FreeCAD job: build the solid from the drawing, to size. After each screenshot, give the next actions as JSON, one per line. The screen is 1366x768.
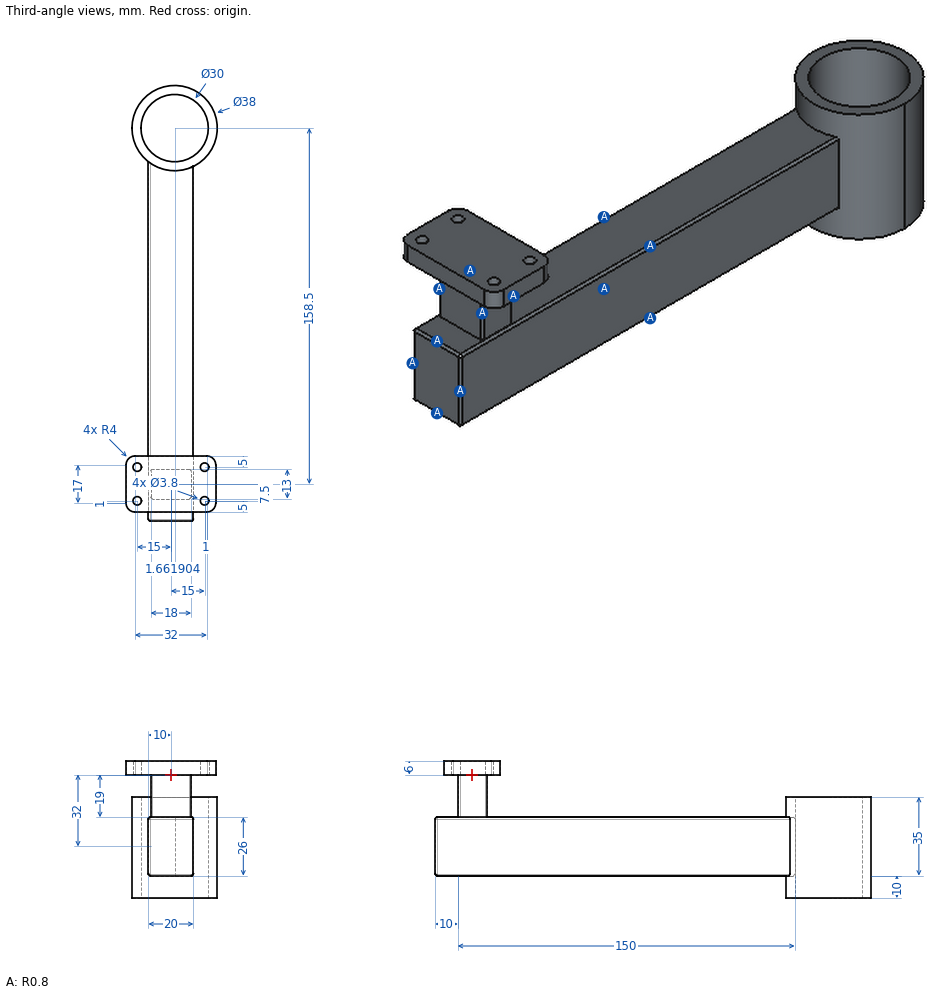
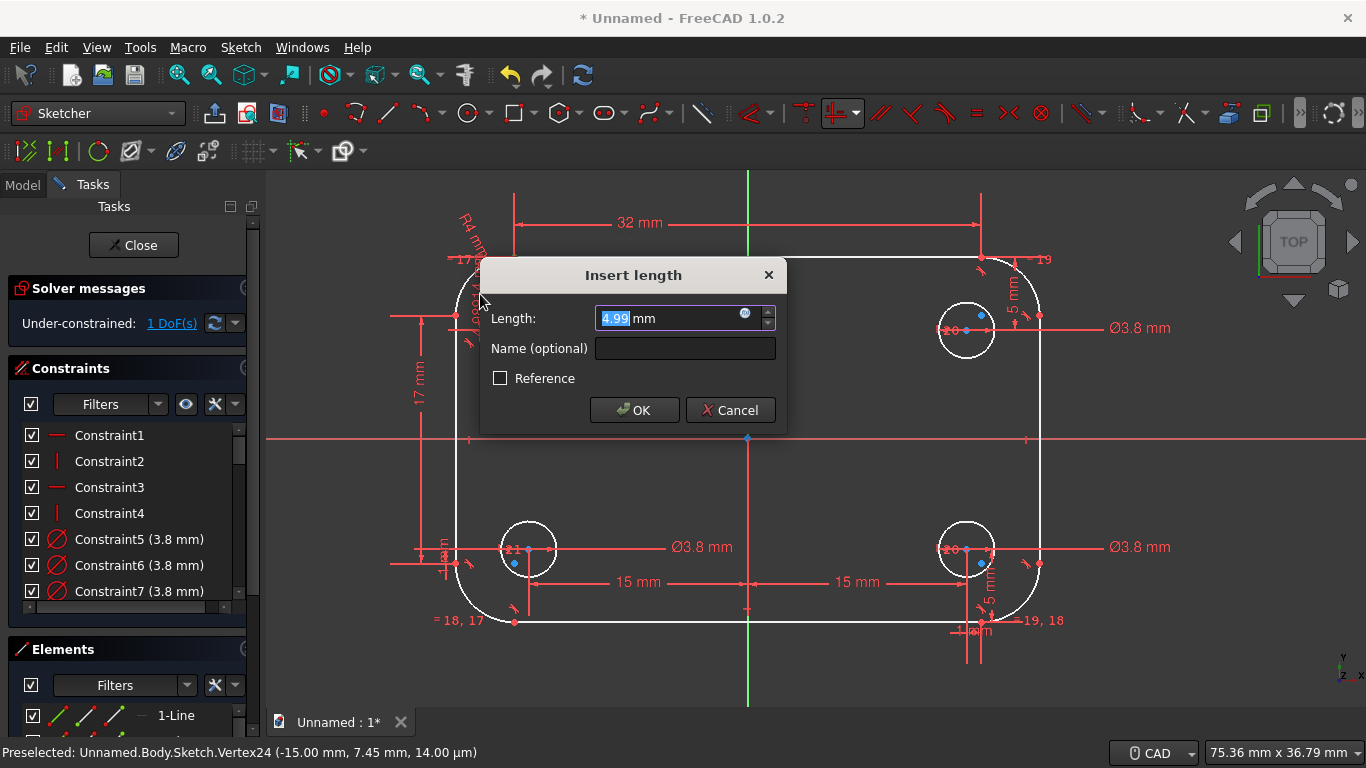
{"action": "type", "text": "5"}
{"action": "key", "text": "Return"}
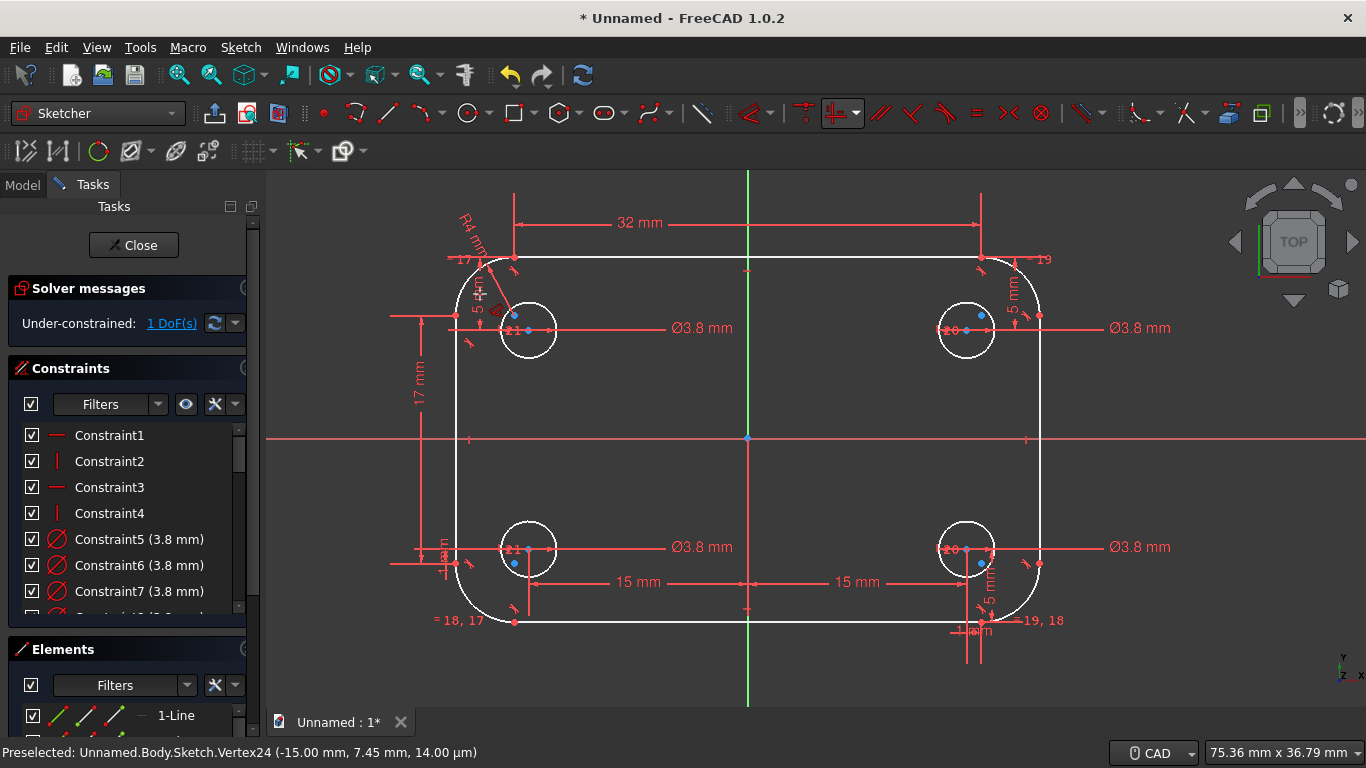
{"action": "left_click", "coordinate": [967, 549]}
{"action": "left_click", "coordinate": [1001, 494]}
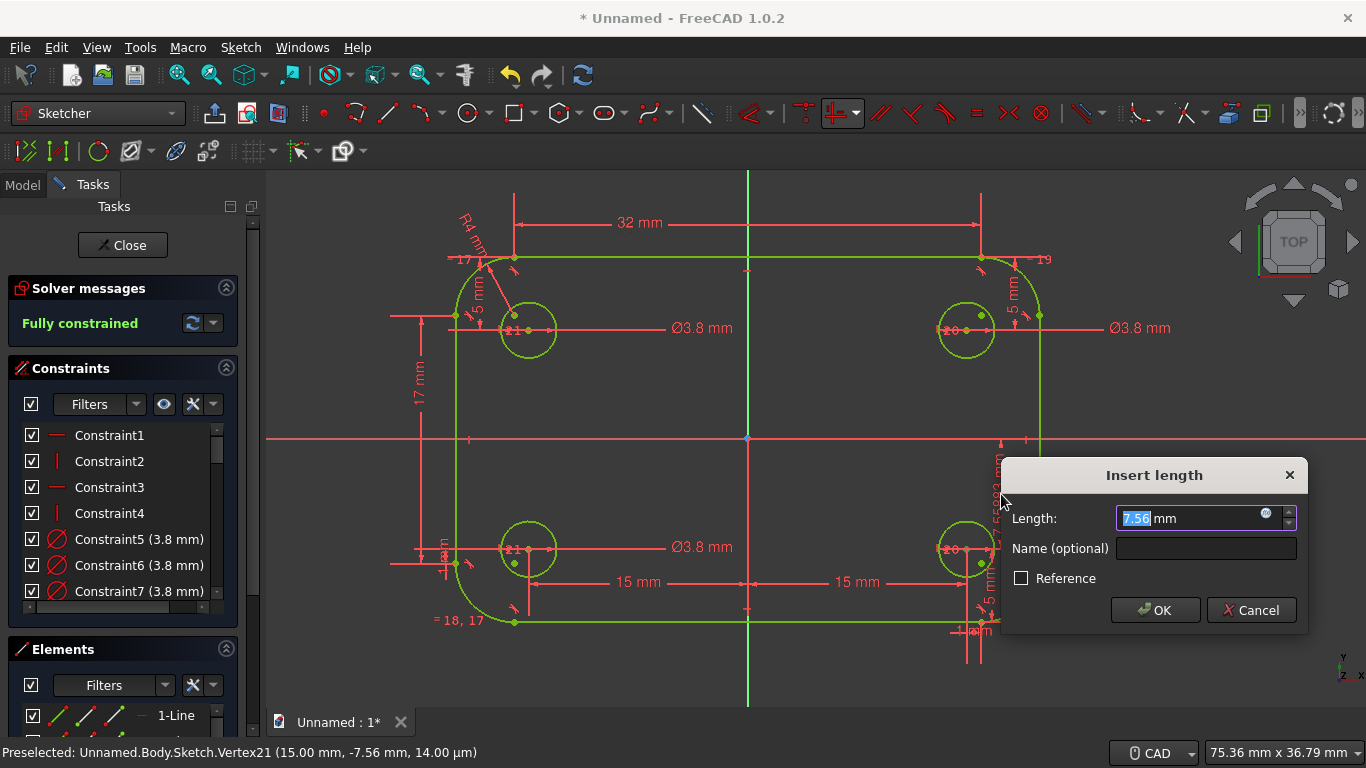
{"action": "type", "text": "7.5"}
{"action": "key", "text": "Return"}
{"action": "key", "text": "Escape"}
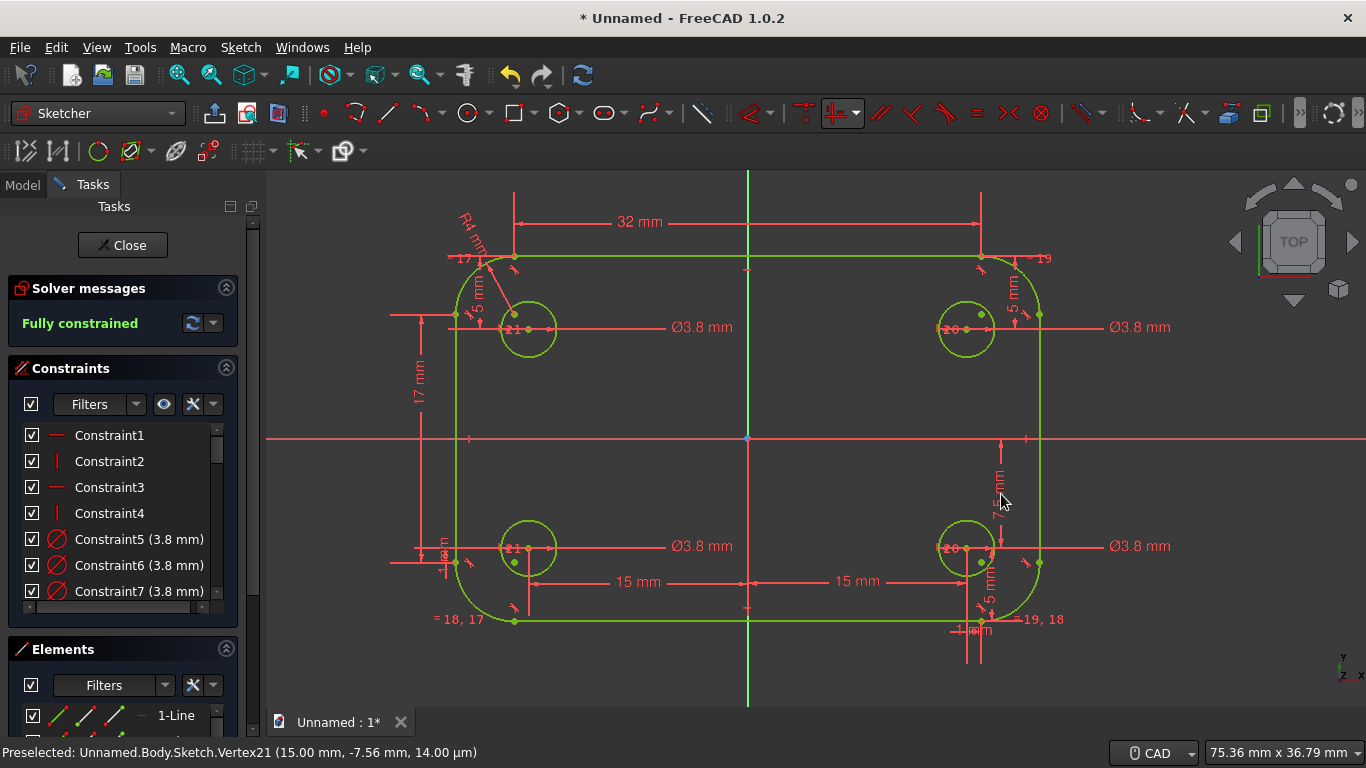
{"action": "left_click", "coordinate": [123, 245]}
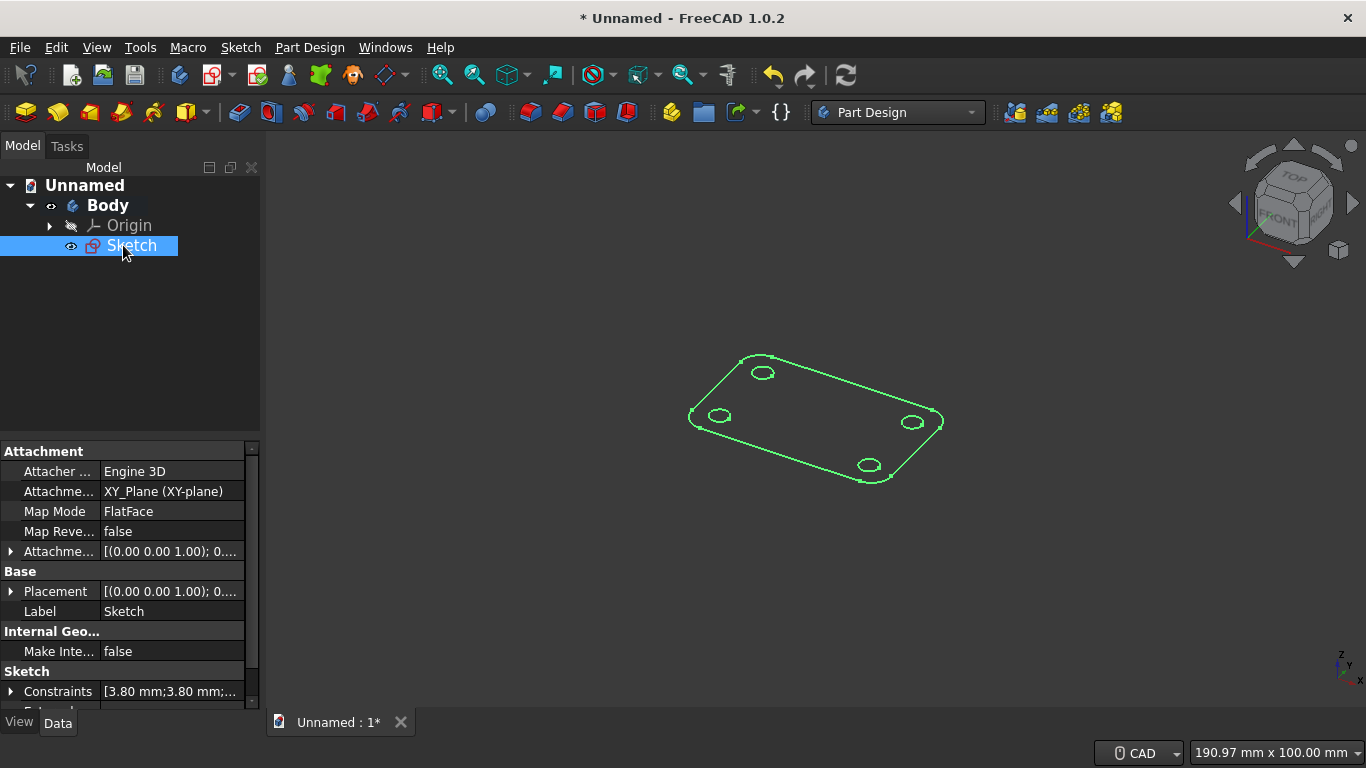
{"action": "left_click", "coordinate": [26, 112]}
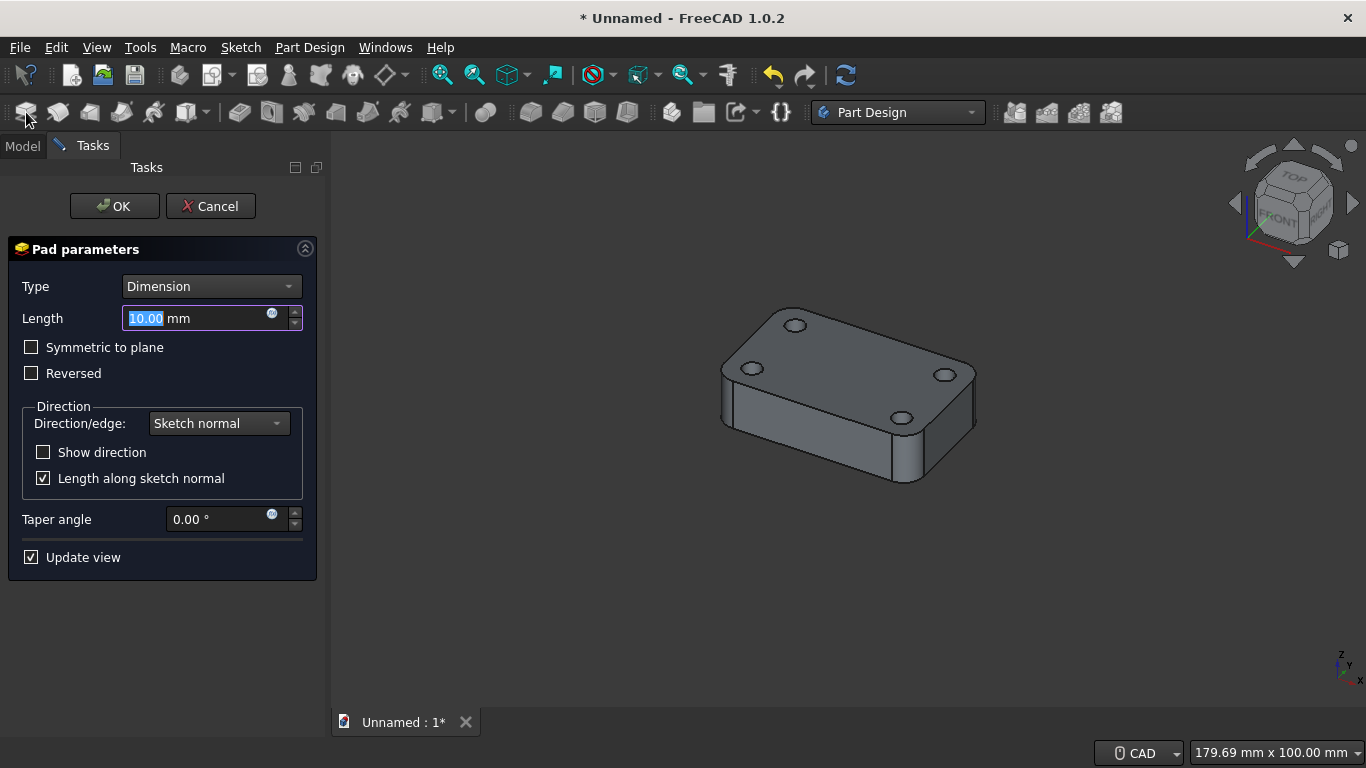
{"action": "type", "text": "6"}
{"action": "key", "text": "Tab"}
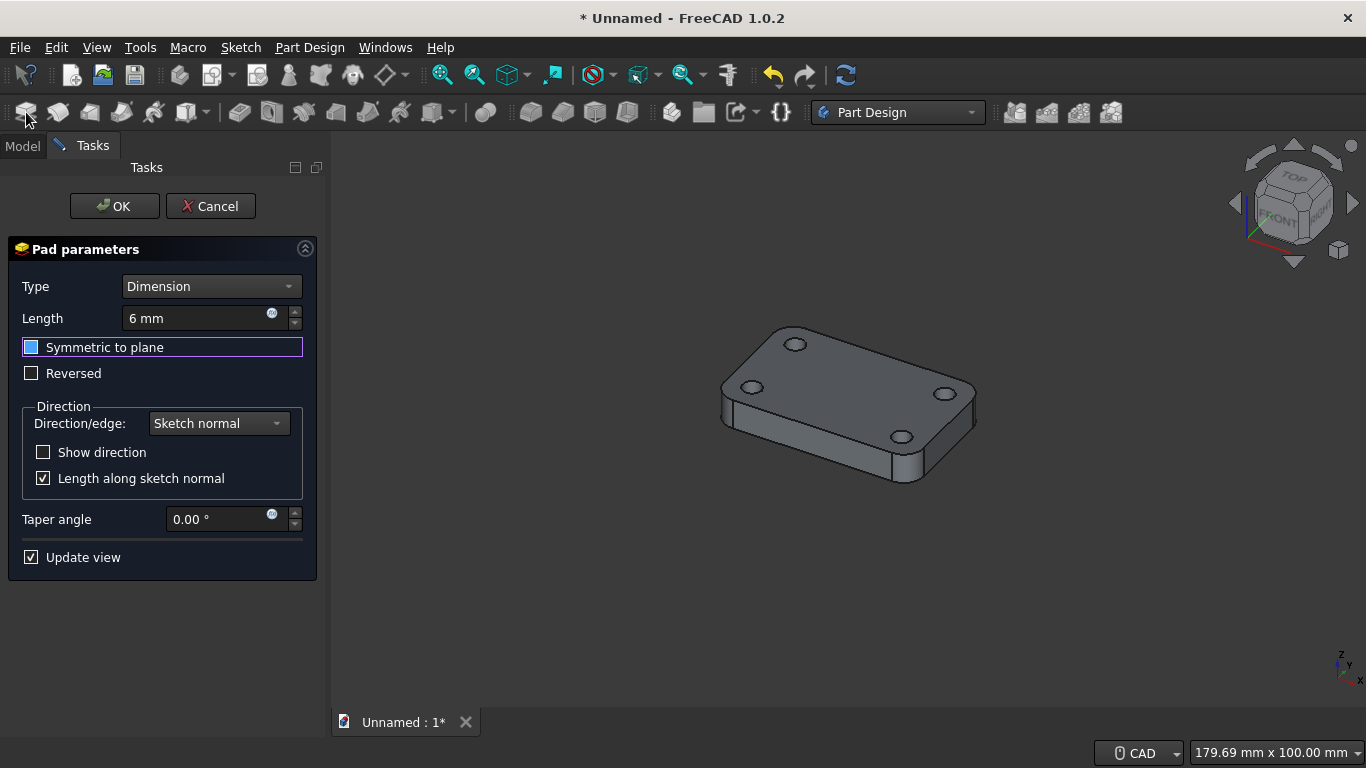
{"action": "left_click", "coordinate": [115, 206]}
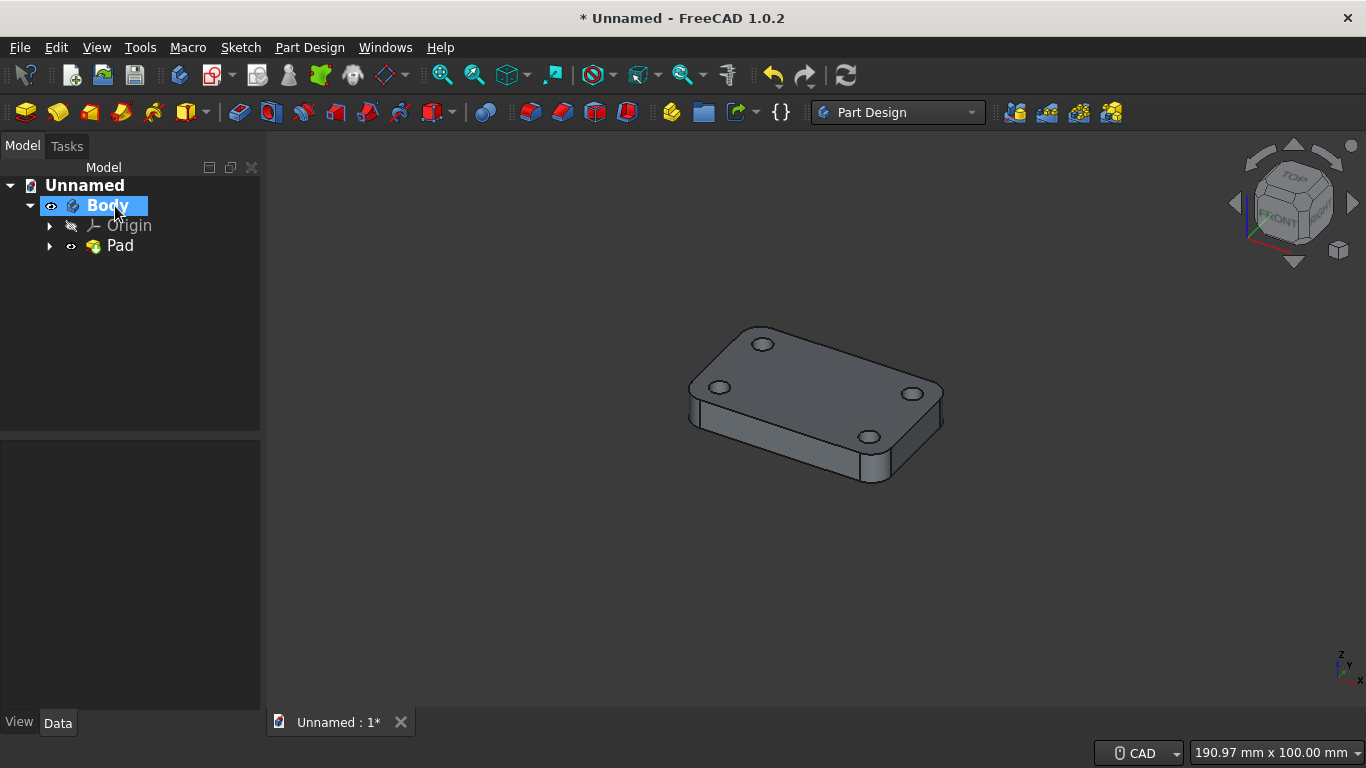
{"action": "left_click", "coordinate": [444, 76]}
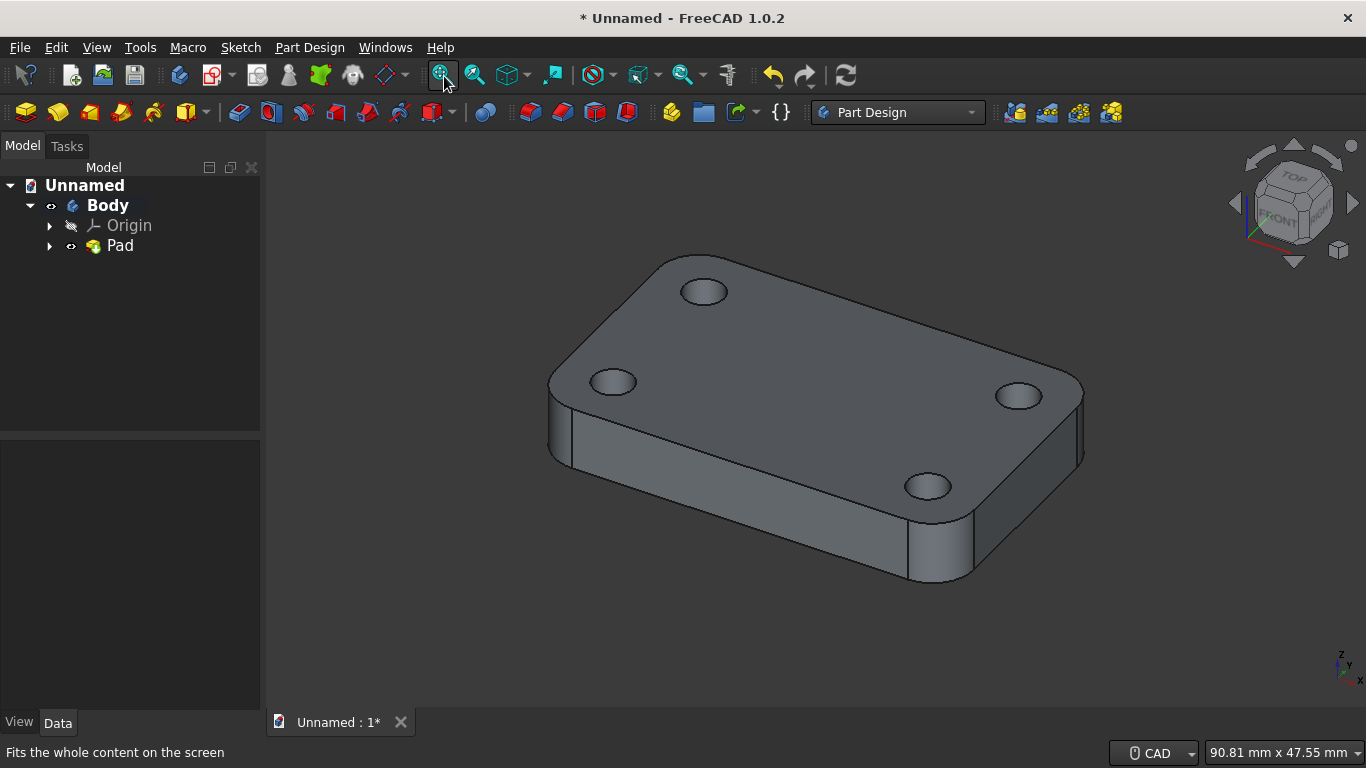
{"action": "left_click", "coordinate": [212, 76]}